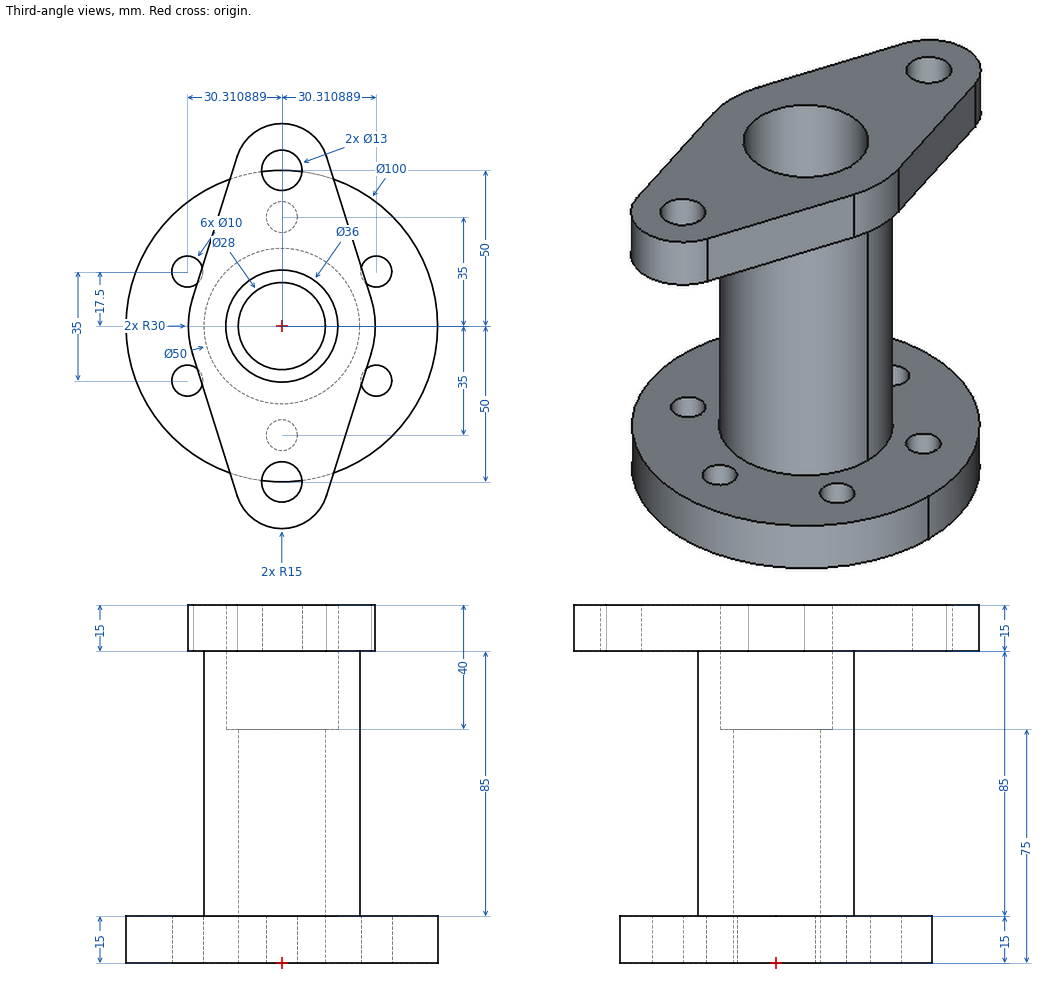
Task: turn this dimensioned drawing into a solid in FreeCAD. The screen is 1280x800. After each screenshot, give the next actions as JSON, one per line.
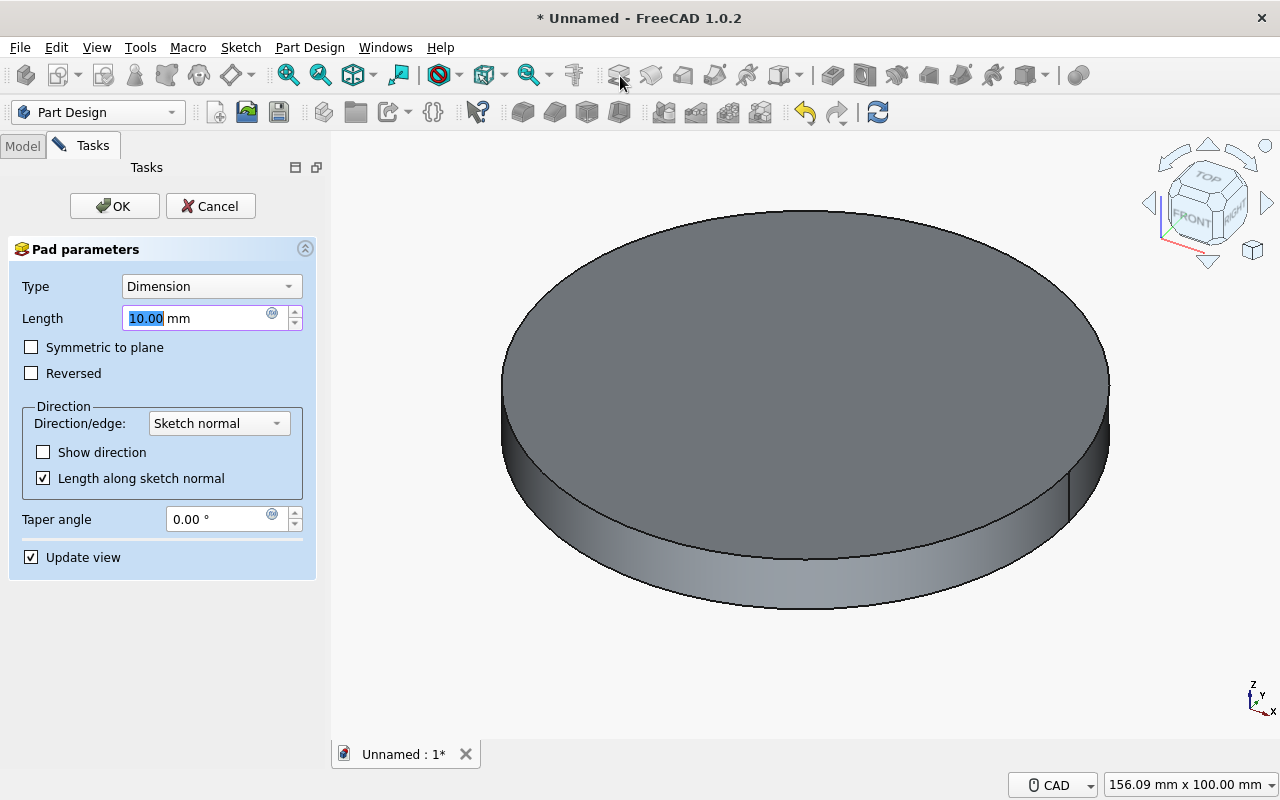
{"action": "type", "text": "15"}
{"action": "key", "text": "Tab"}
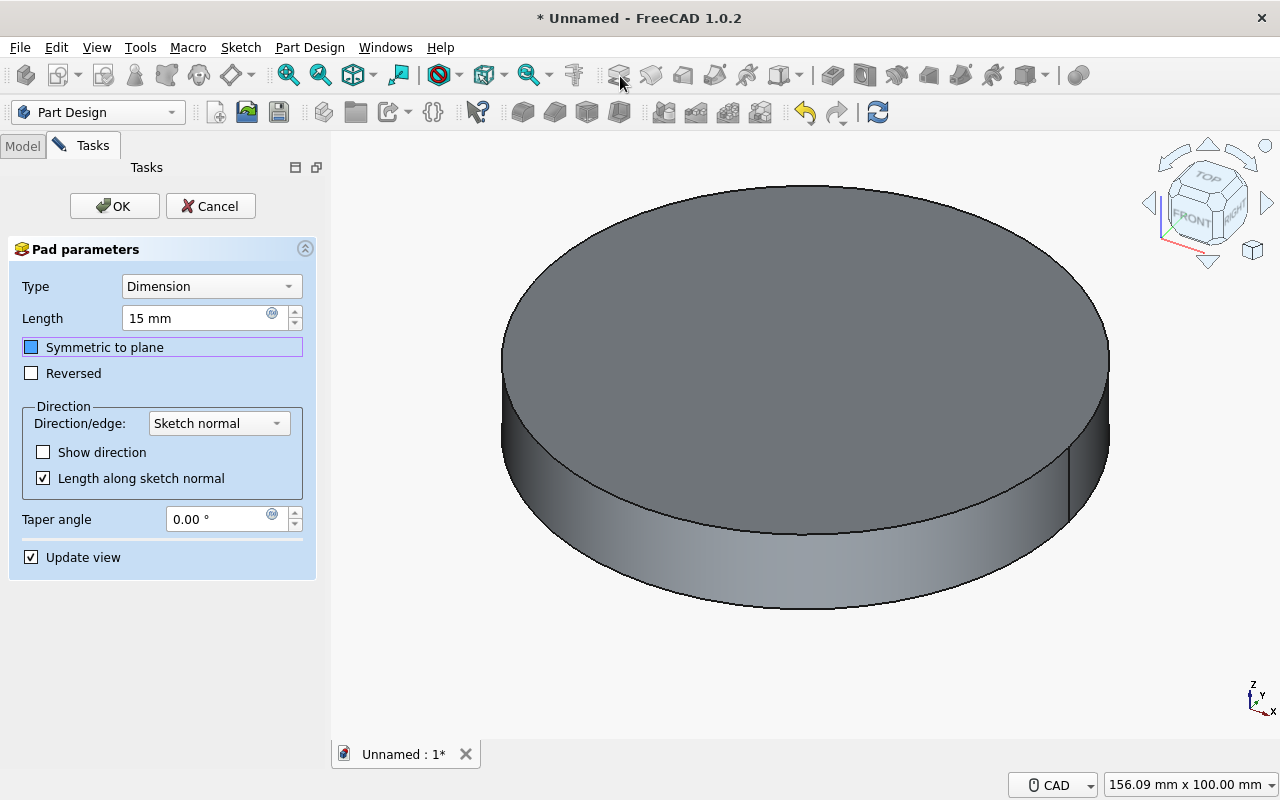
{"action": "left_click", "coordinate": [115, 206]}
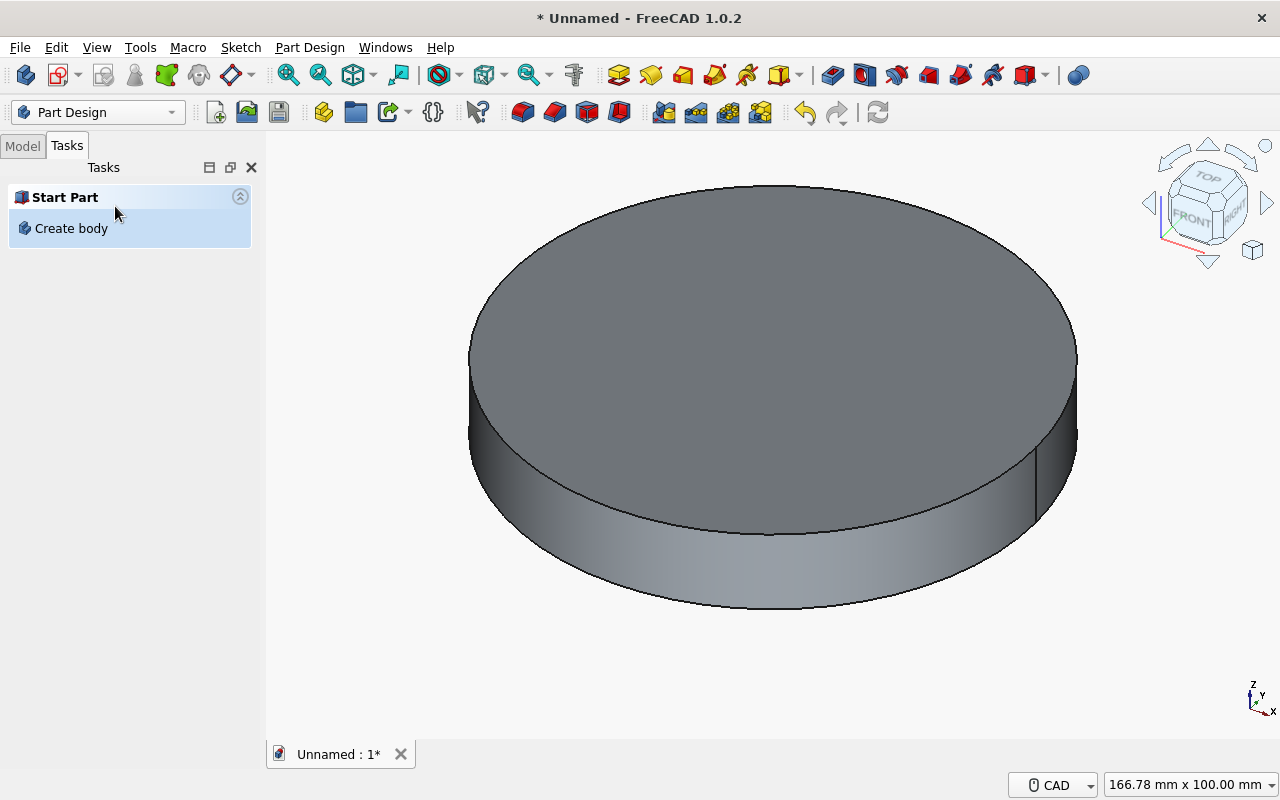
{"action": "key", "text": "v f"}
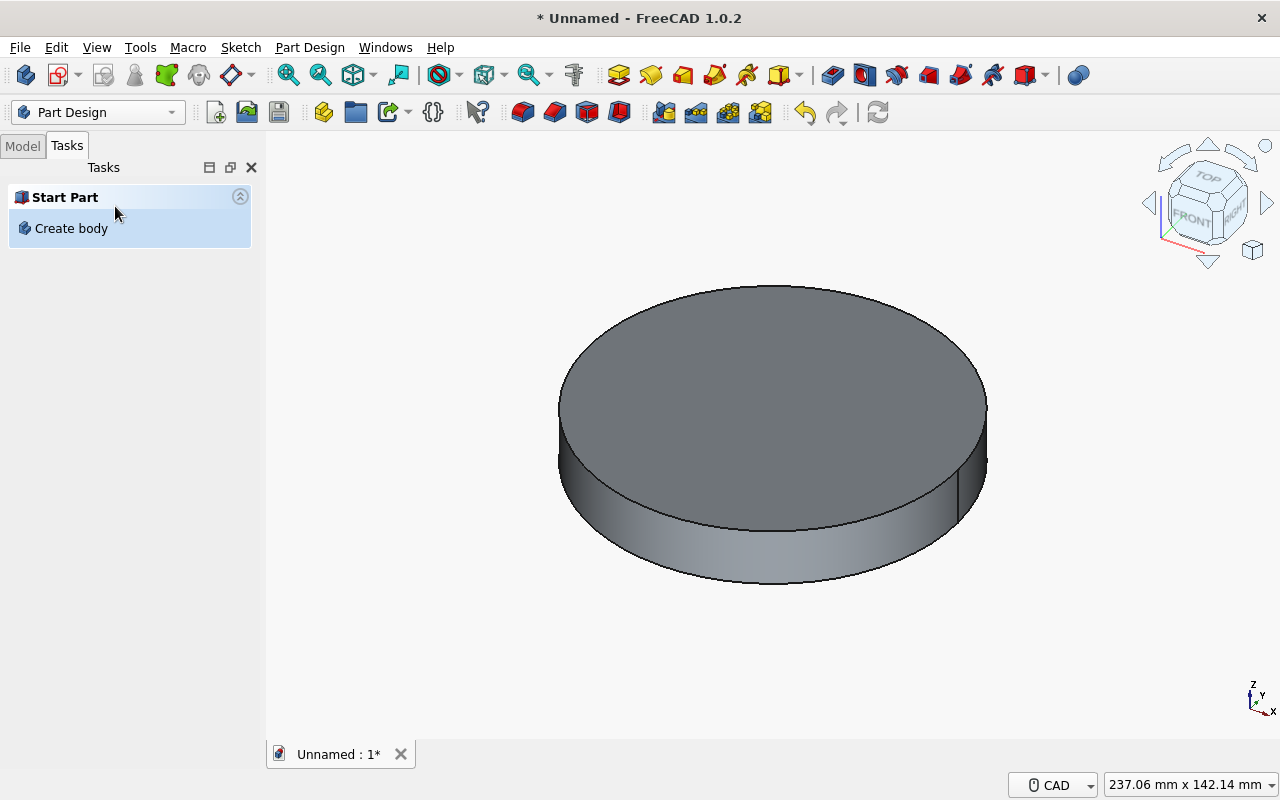
{"action": "left_click", "coordinate": [773, 408]}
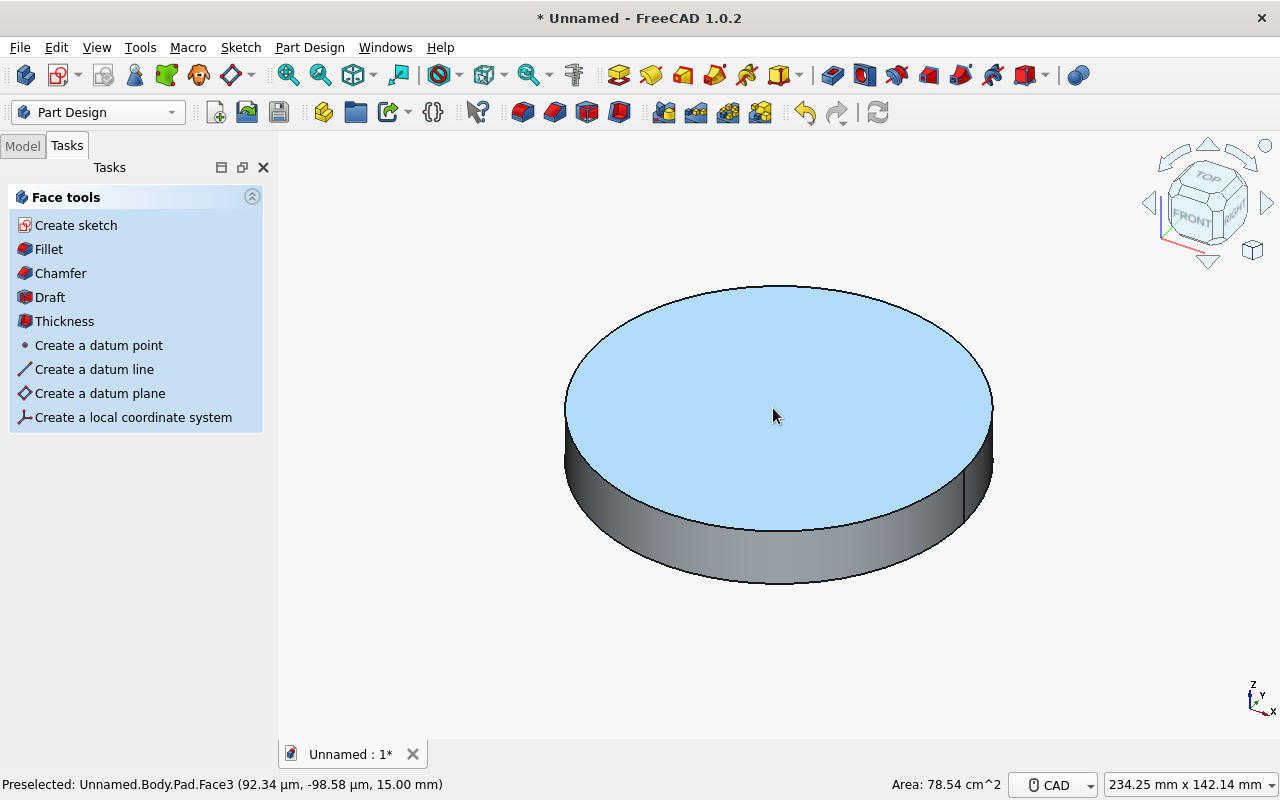
{"action": "left_click", "coordinate": [58, 76]}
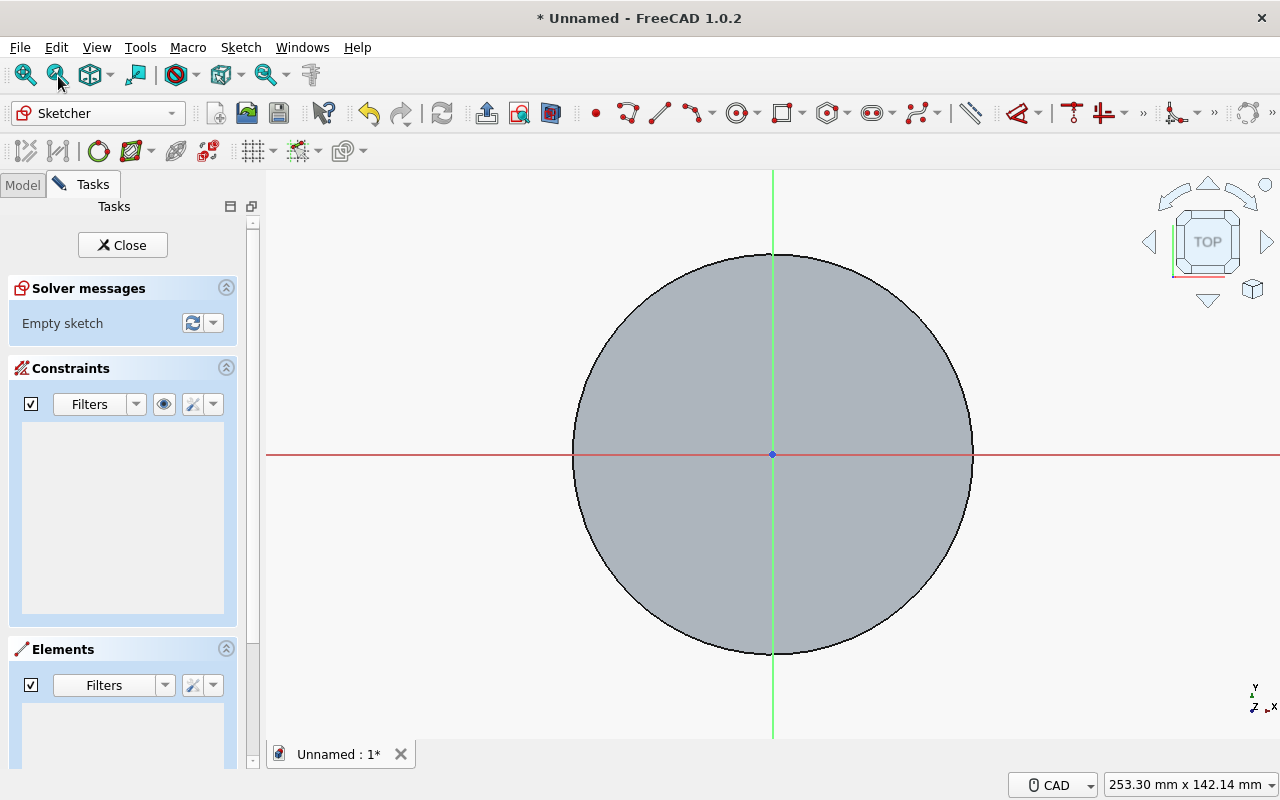
{"action": "left_click", "coordinate": [738, 114]}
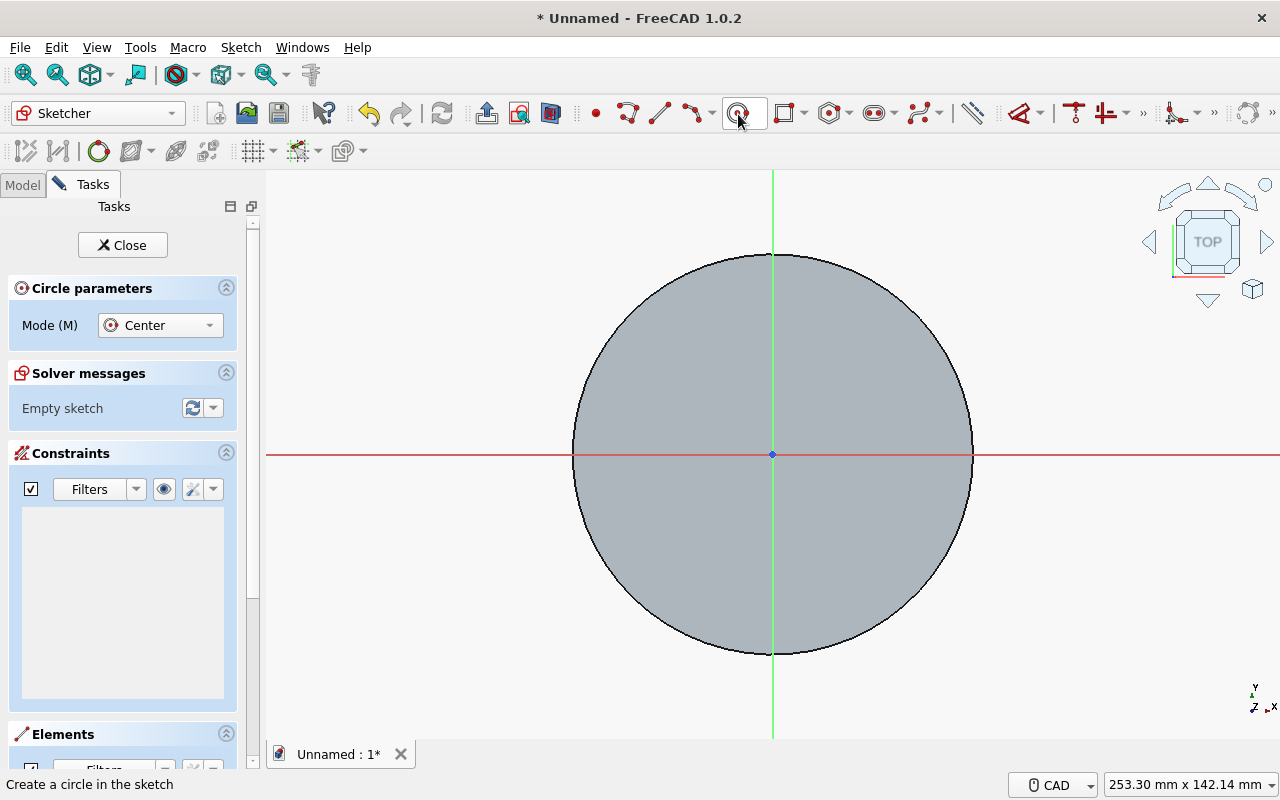
{"action": "left_click", "coordinate": [652, 384]}
{"action": "mouse_move", "coordinate": [666, 370]}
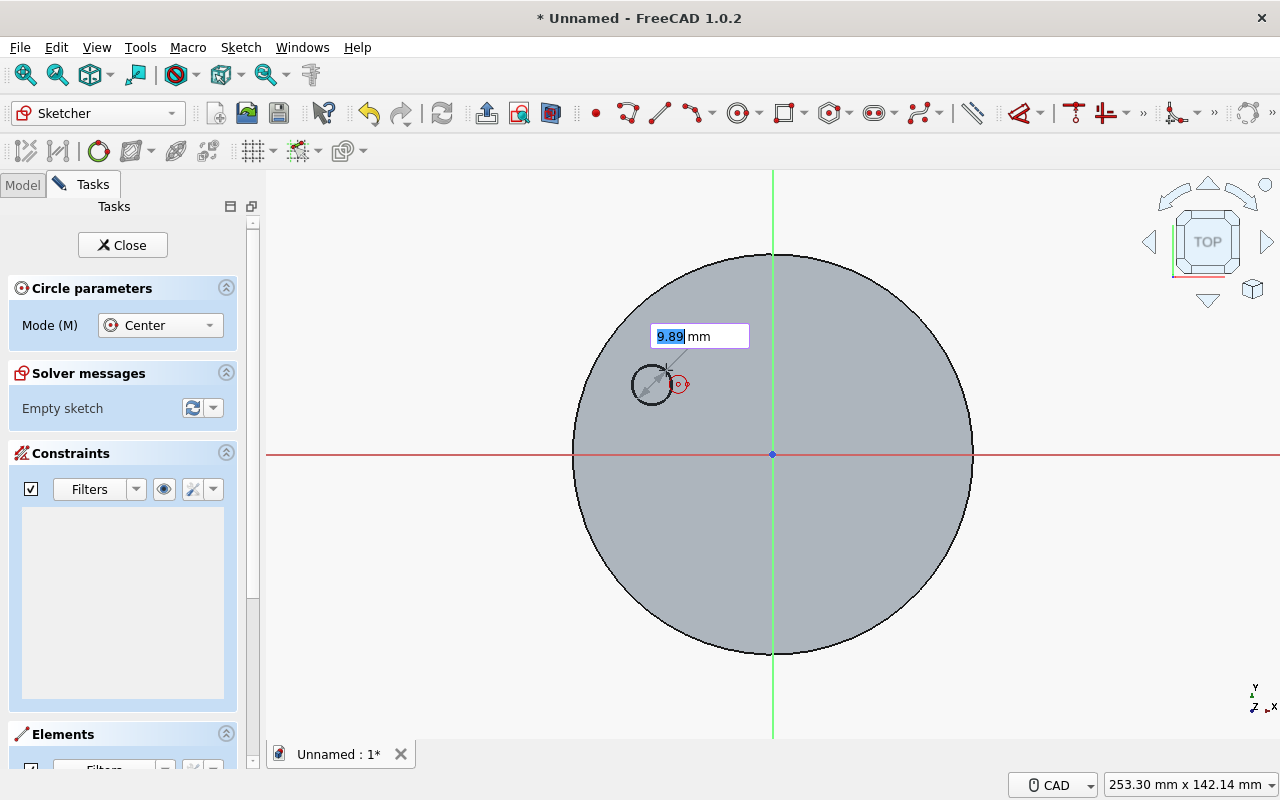
{"action": "type", "text": "10"}
{"action": "key", "text": "Return"}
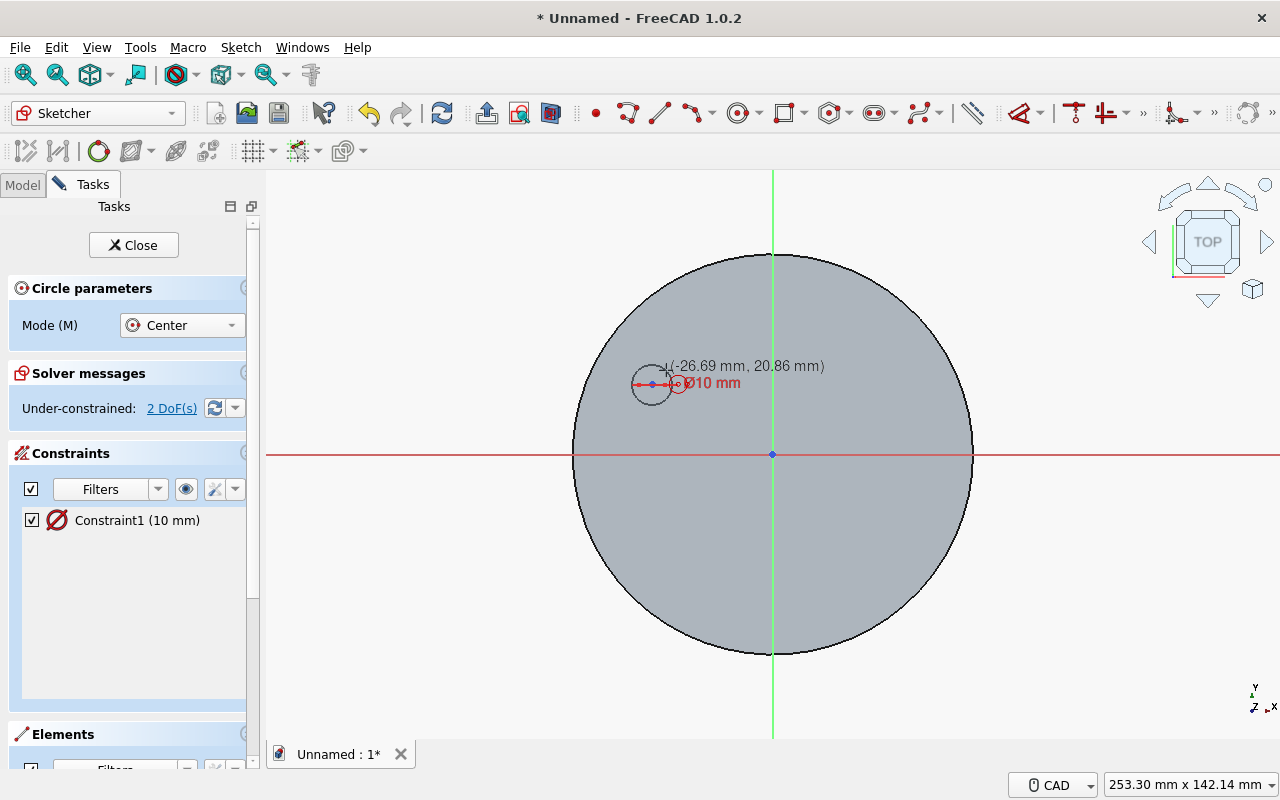
{"action": "left_click", "coordinate": [773, 314]}
{"action": "mouse_move", "coordinate": [787, 300]}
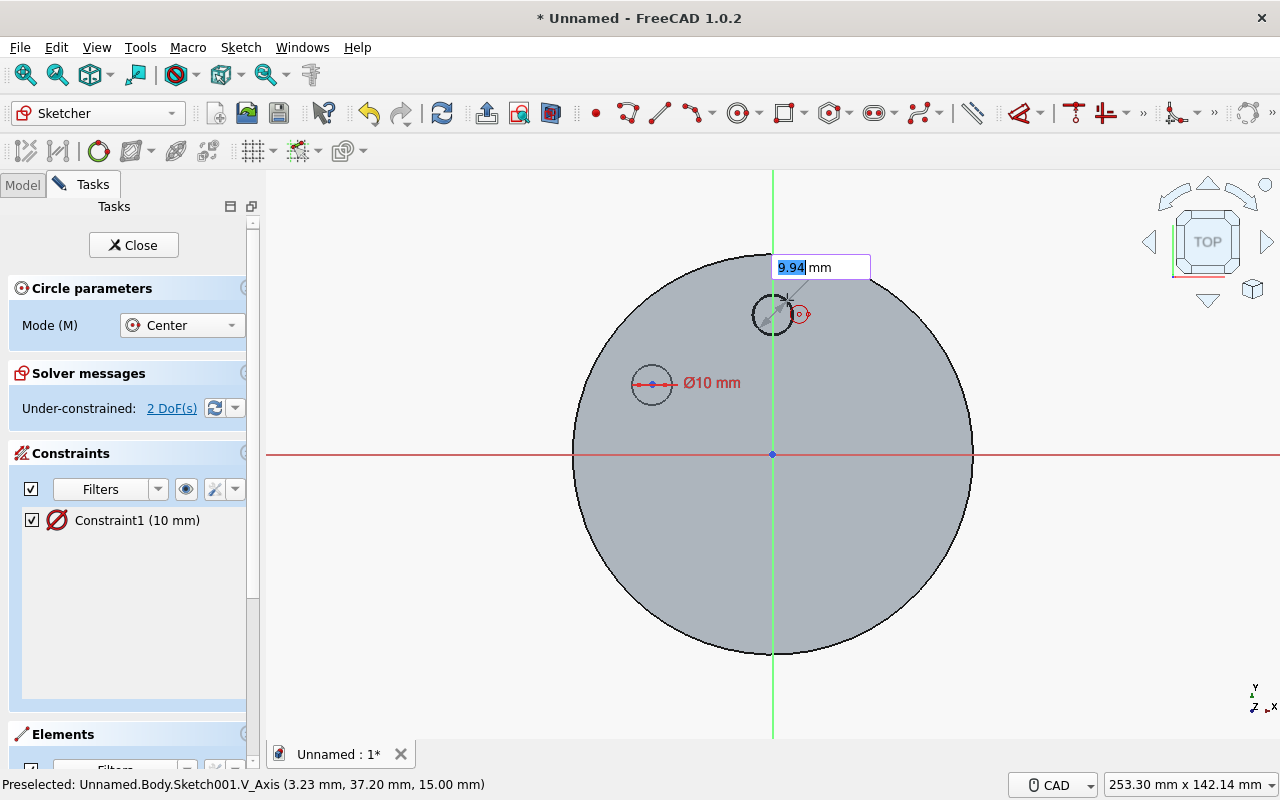
{"action": "type", "text": "10"}
{"action": "key", "text": "Return"}